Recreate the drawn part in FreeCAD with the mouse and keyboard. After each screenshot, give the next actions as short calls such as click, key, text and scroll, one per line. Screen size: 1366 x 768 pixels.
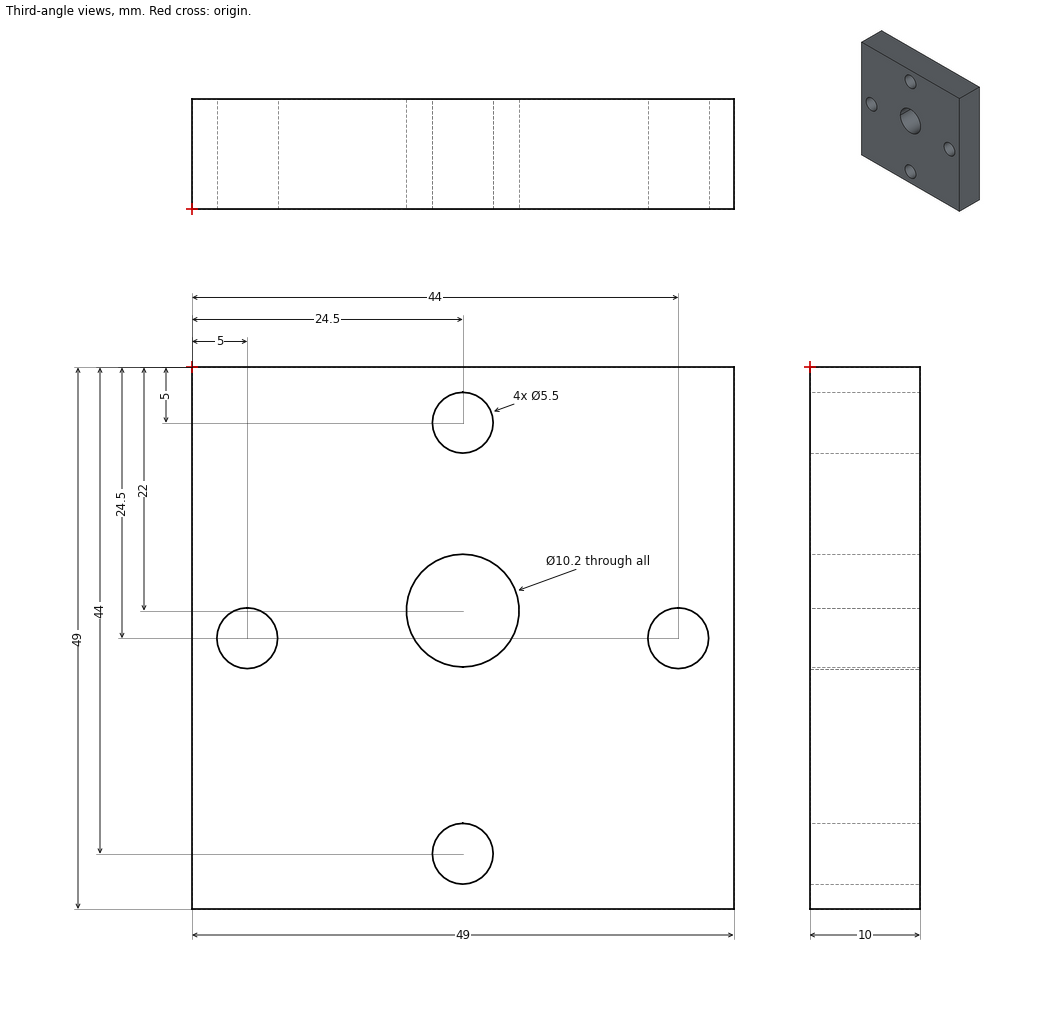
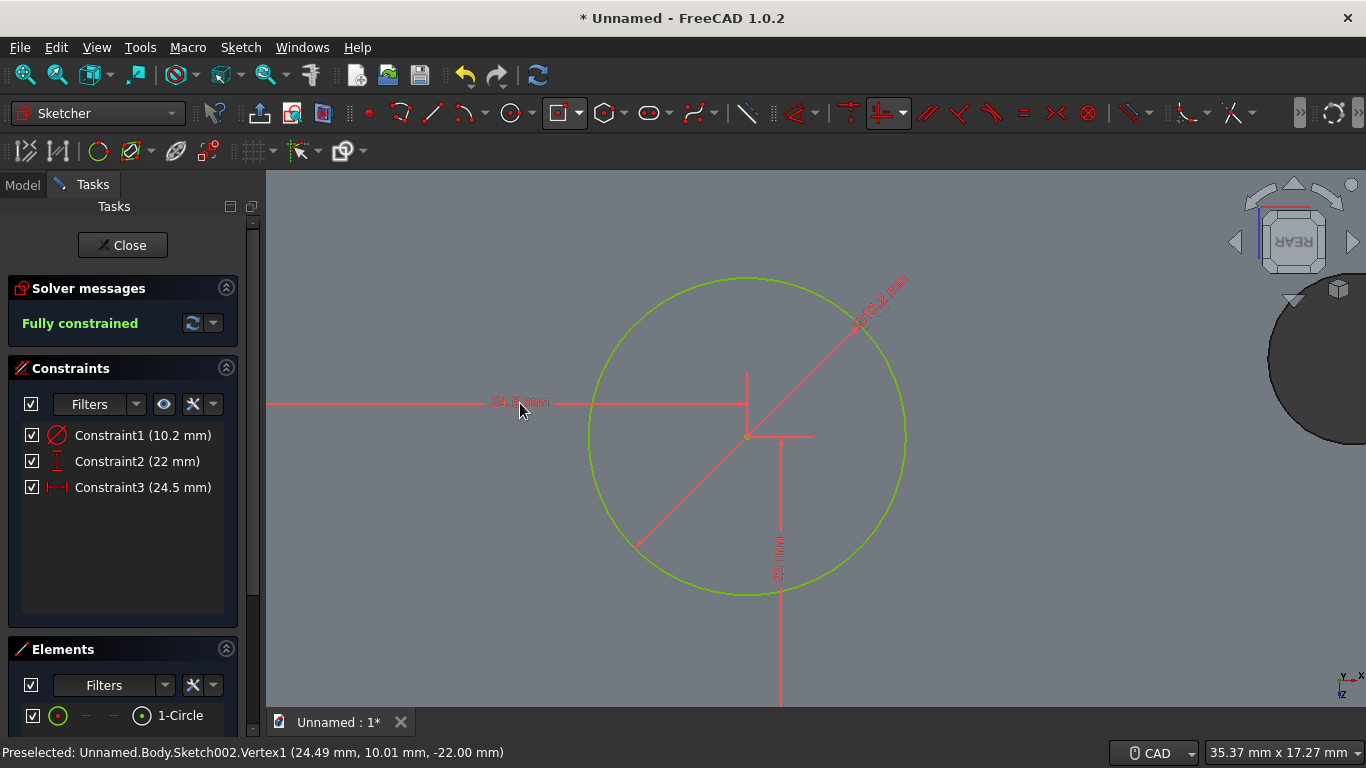
click(123, 245)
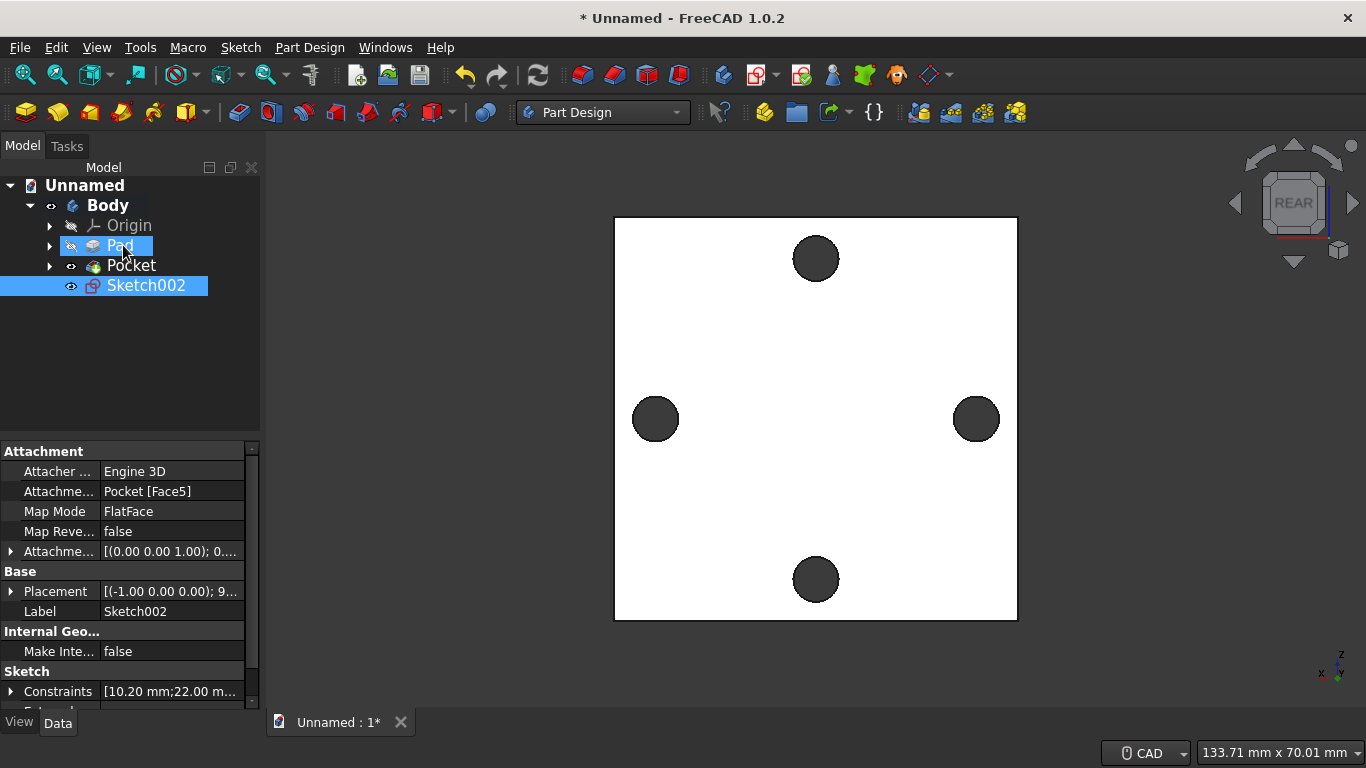
click(272, 112)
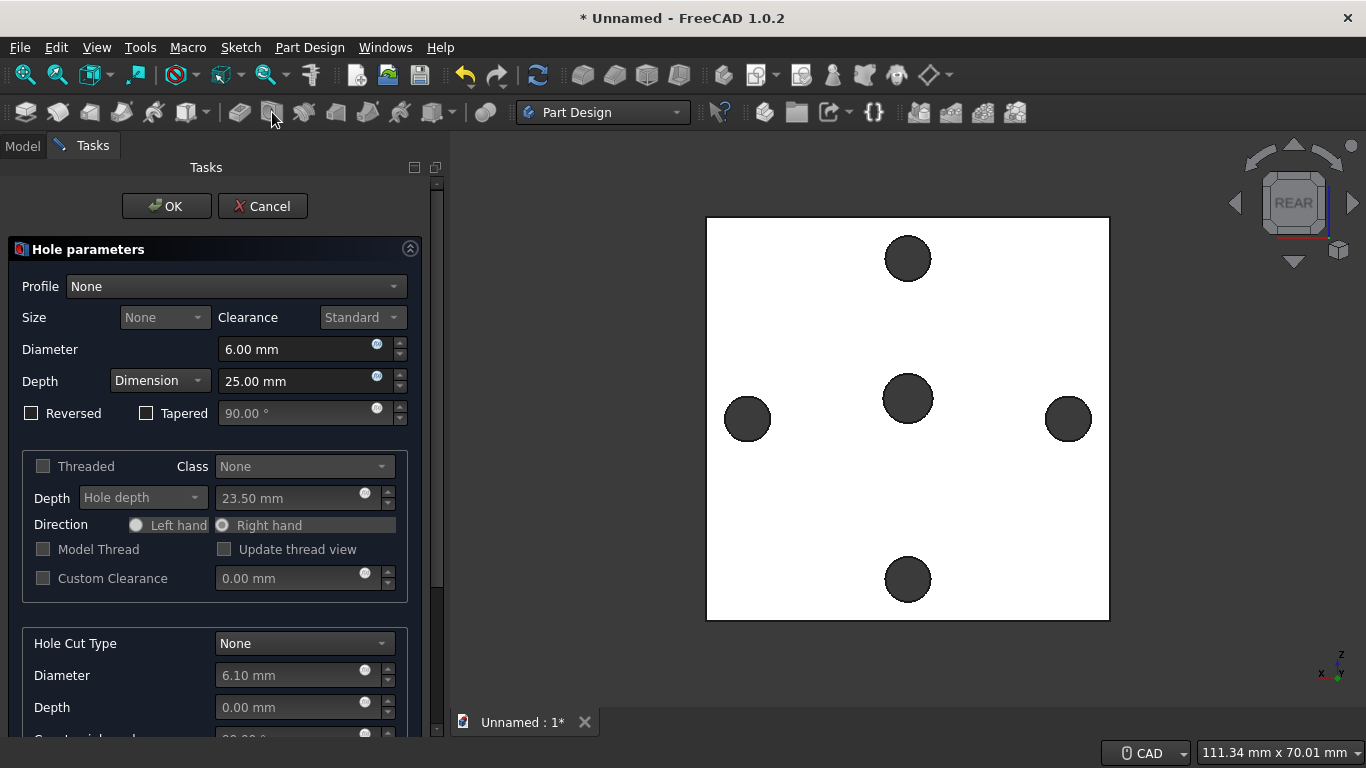
triple_click(305, 349)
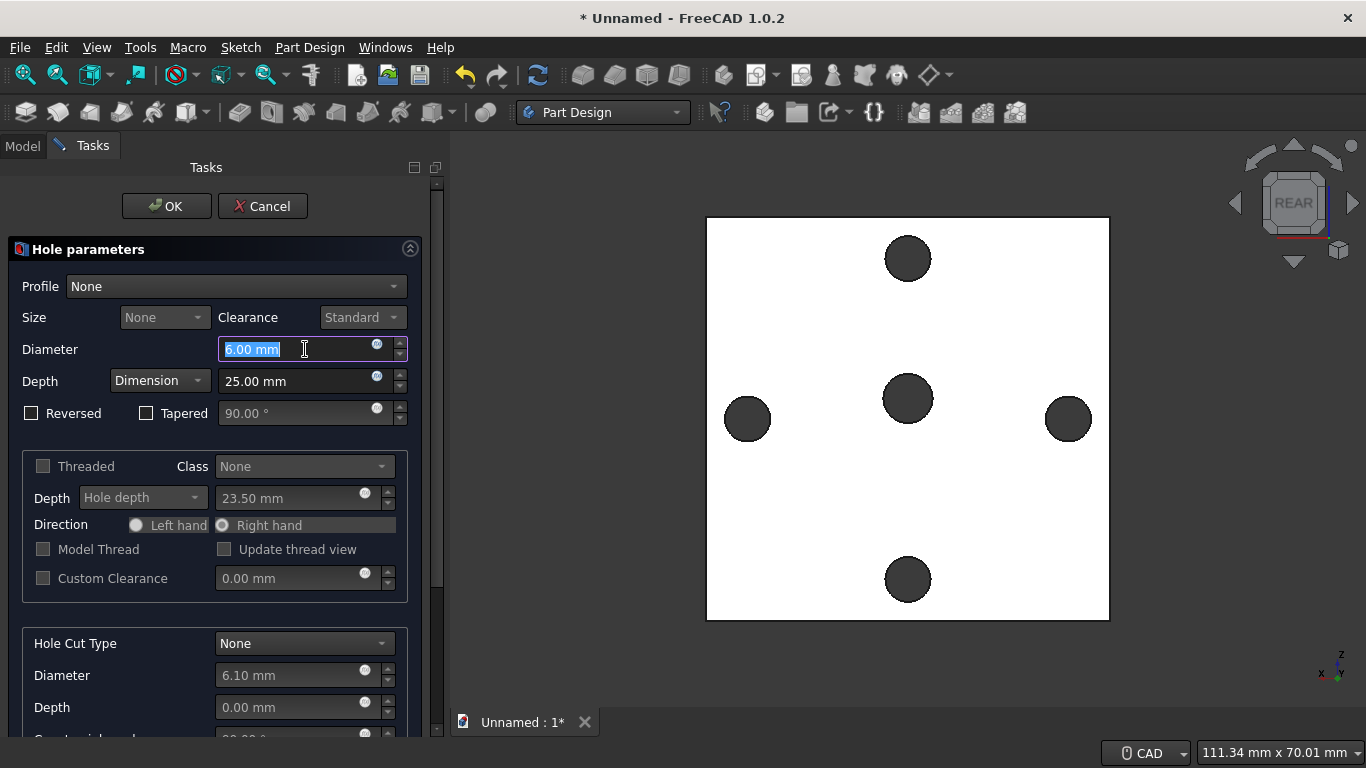
text(10.2)
key(Tab)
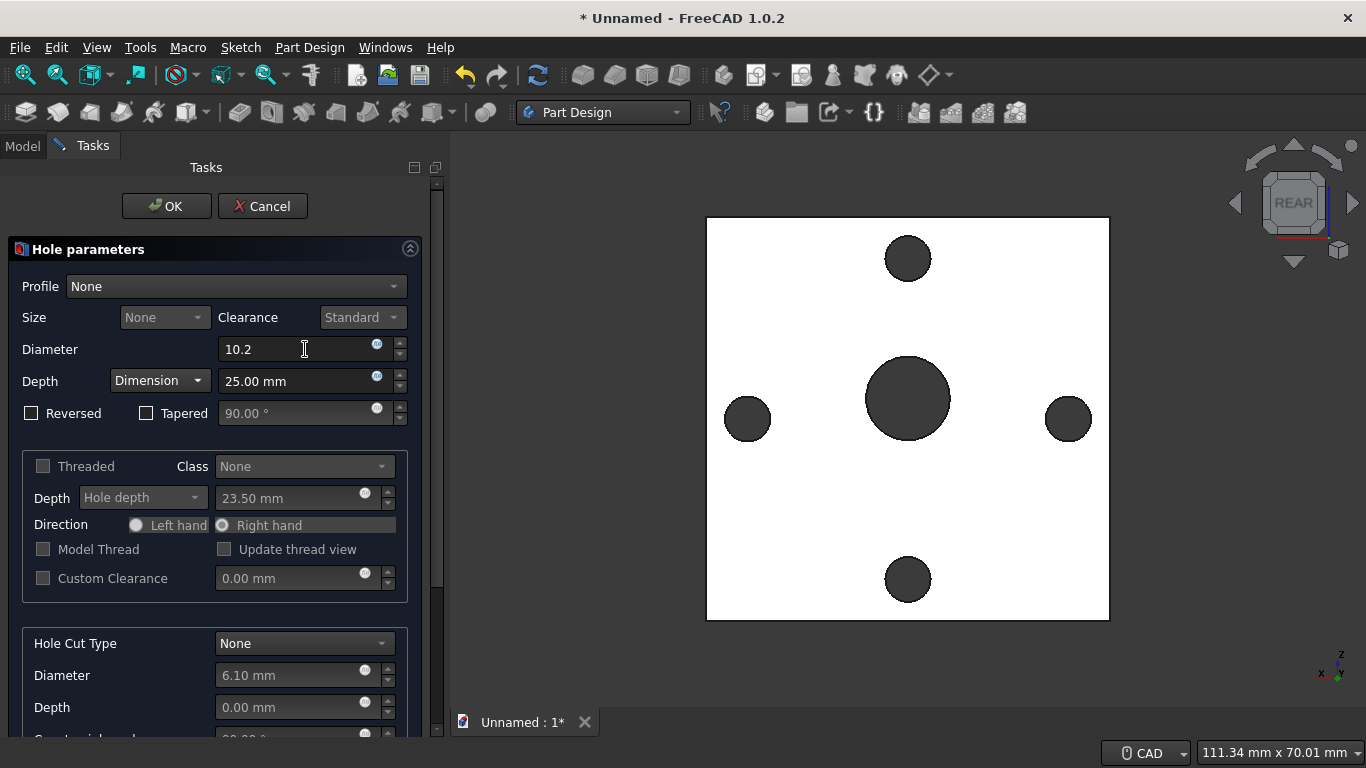
click(161, 380)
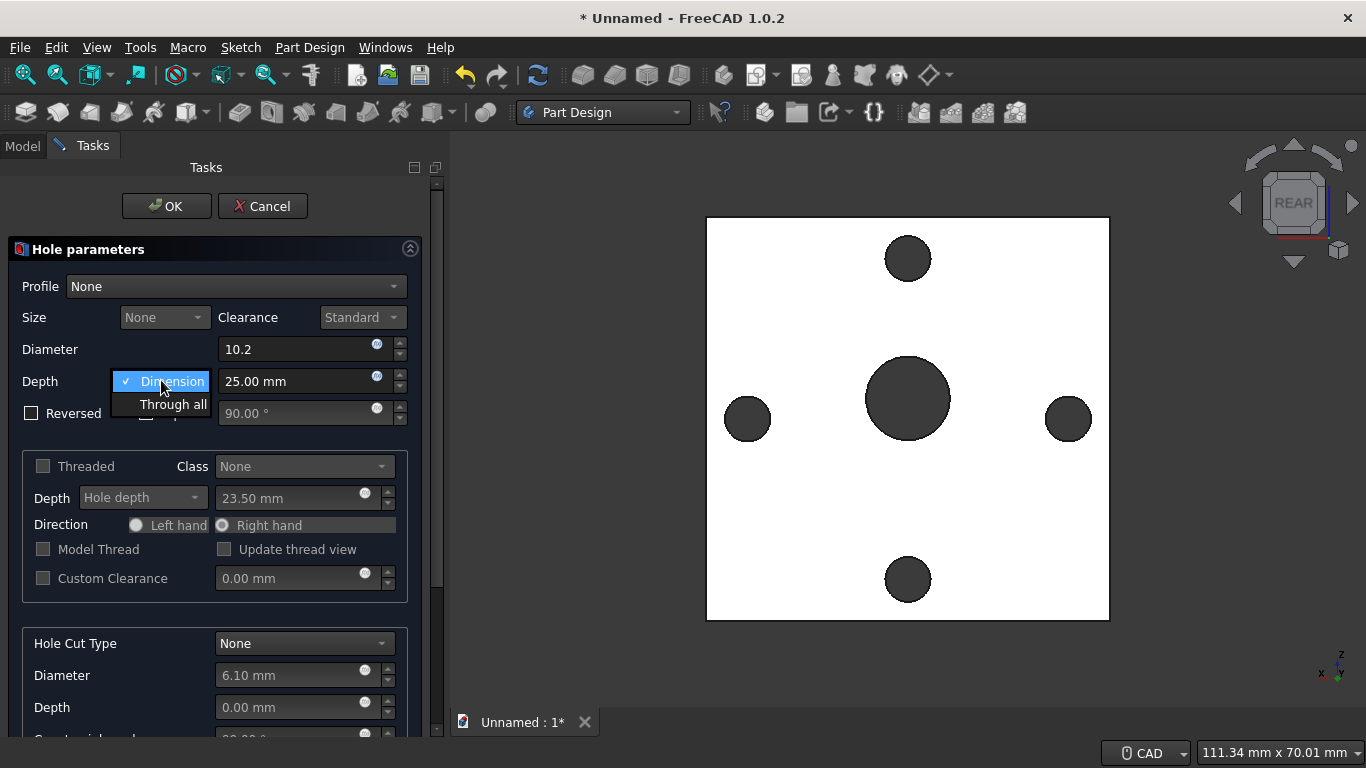
click(160, 404)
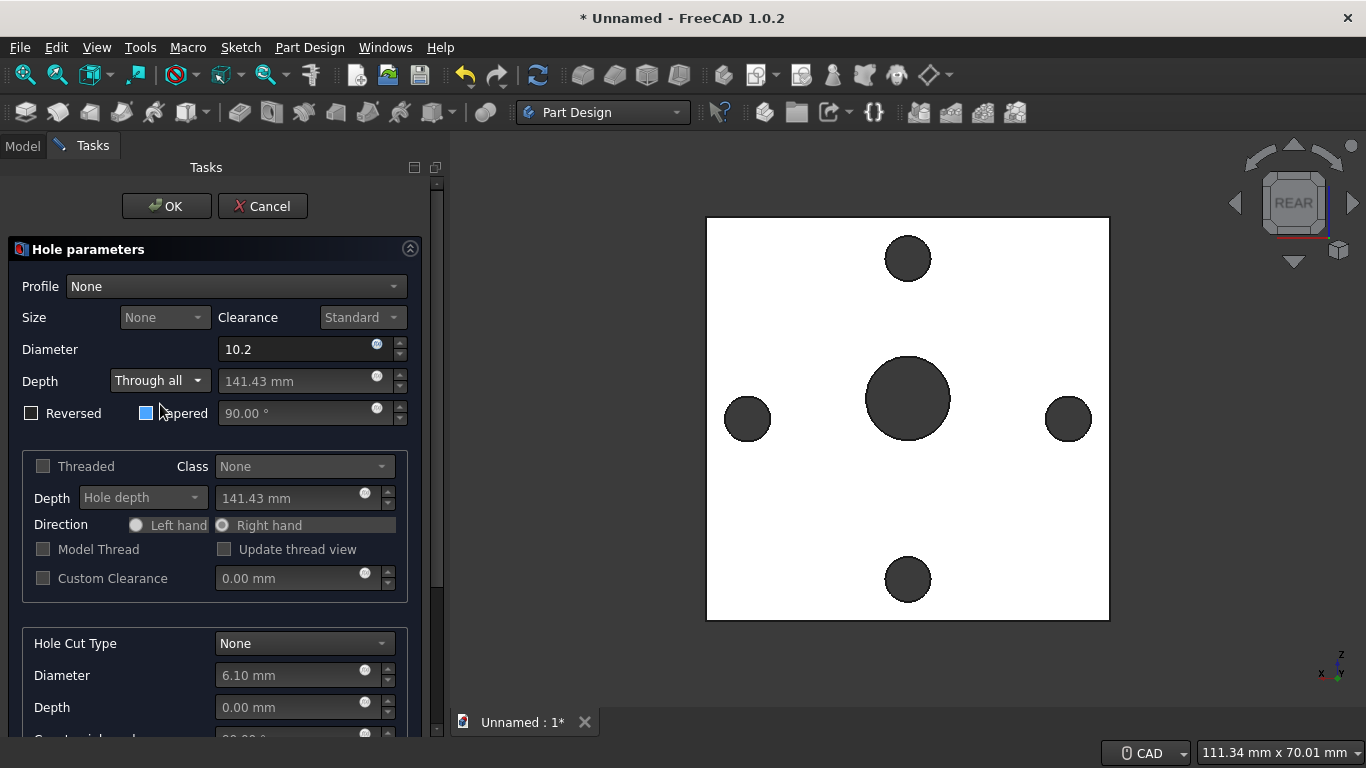
click(167, 206)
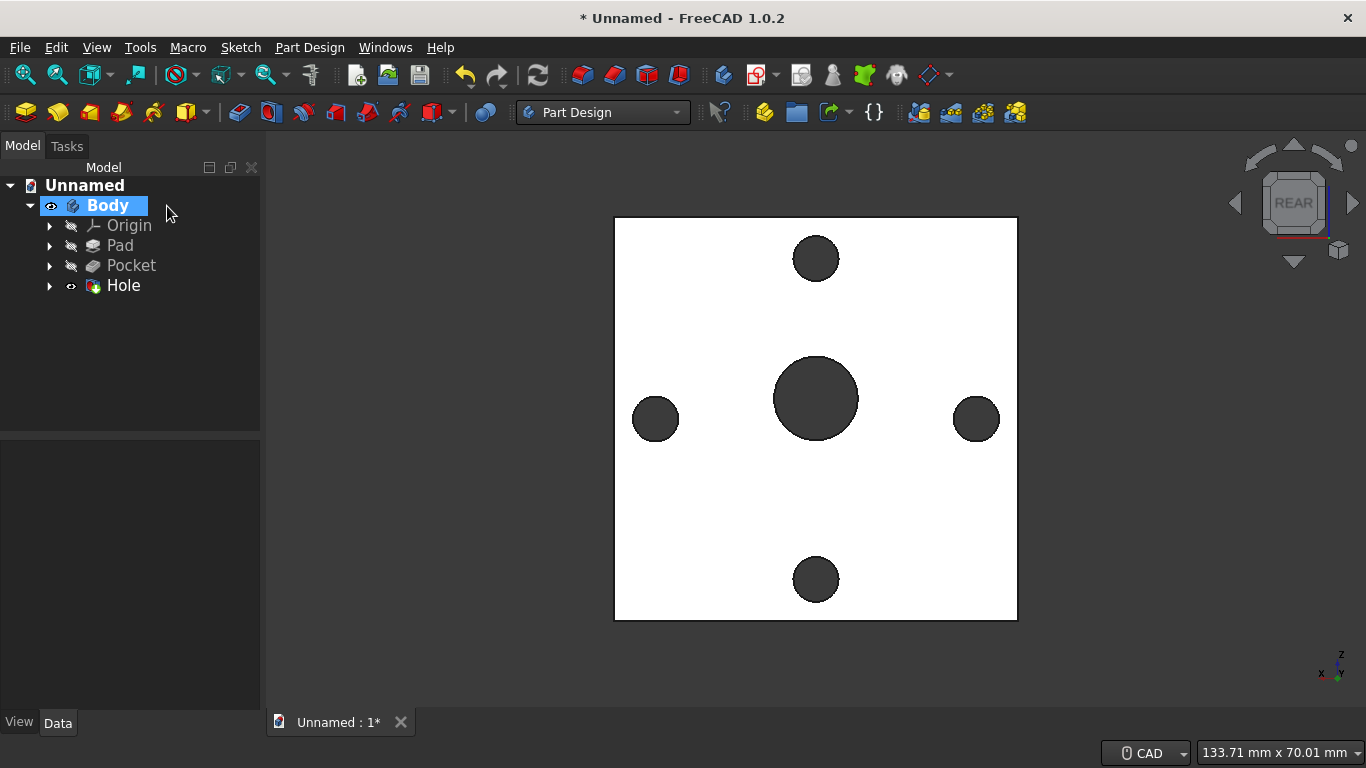
key(0)